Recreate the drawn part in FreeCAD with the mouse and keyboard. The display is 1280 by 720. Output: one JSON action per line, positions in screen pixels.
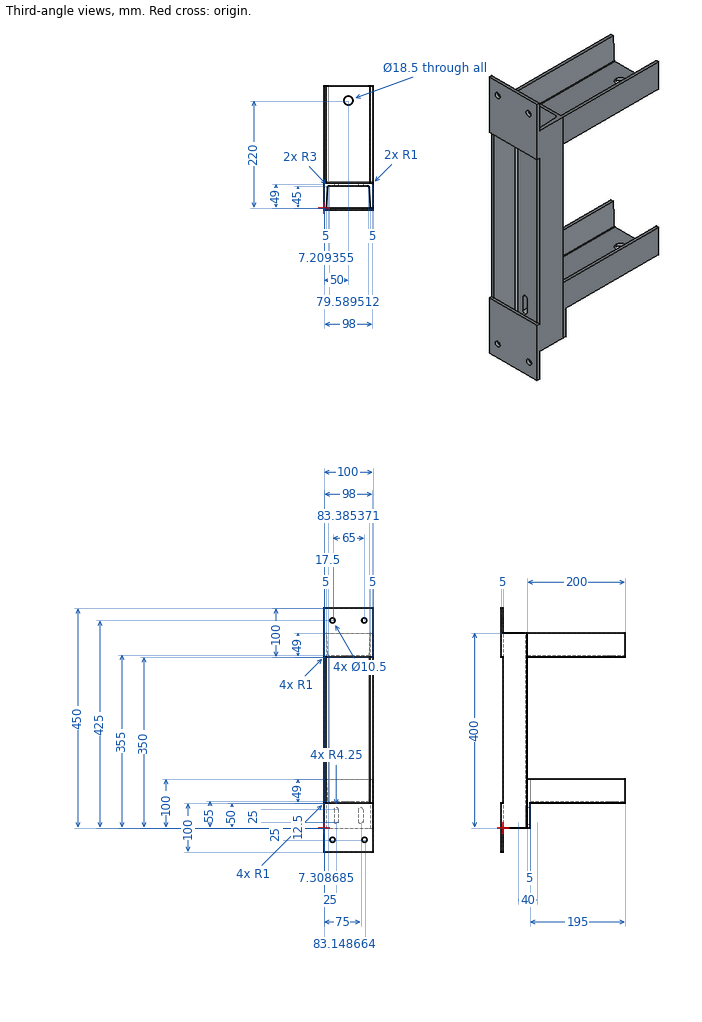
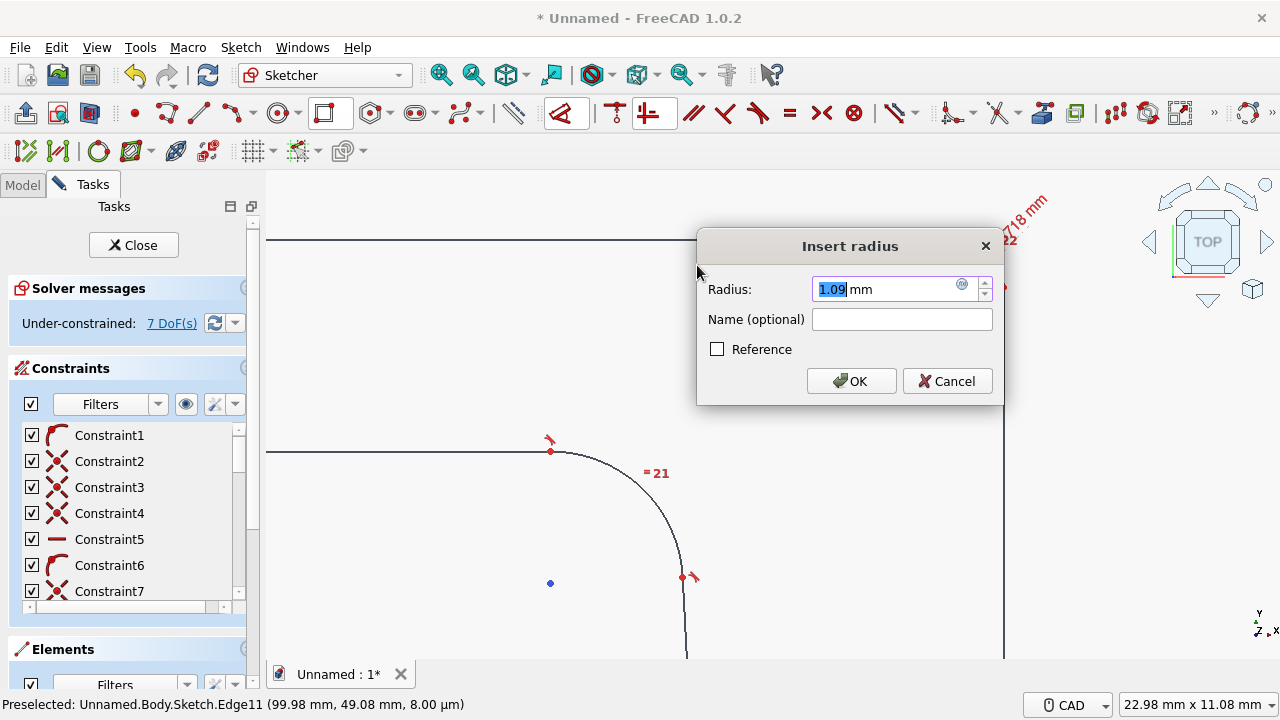
{"action": "type", "text": "1"}
{"action": "key", "text": "Return"}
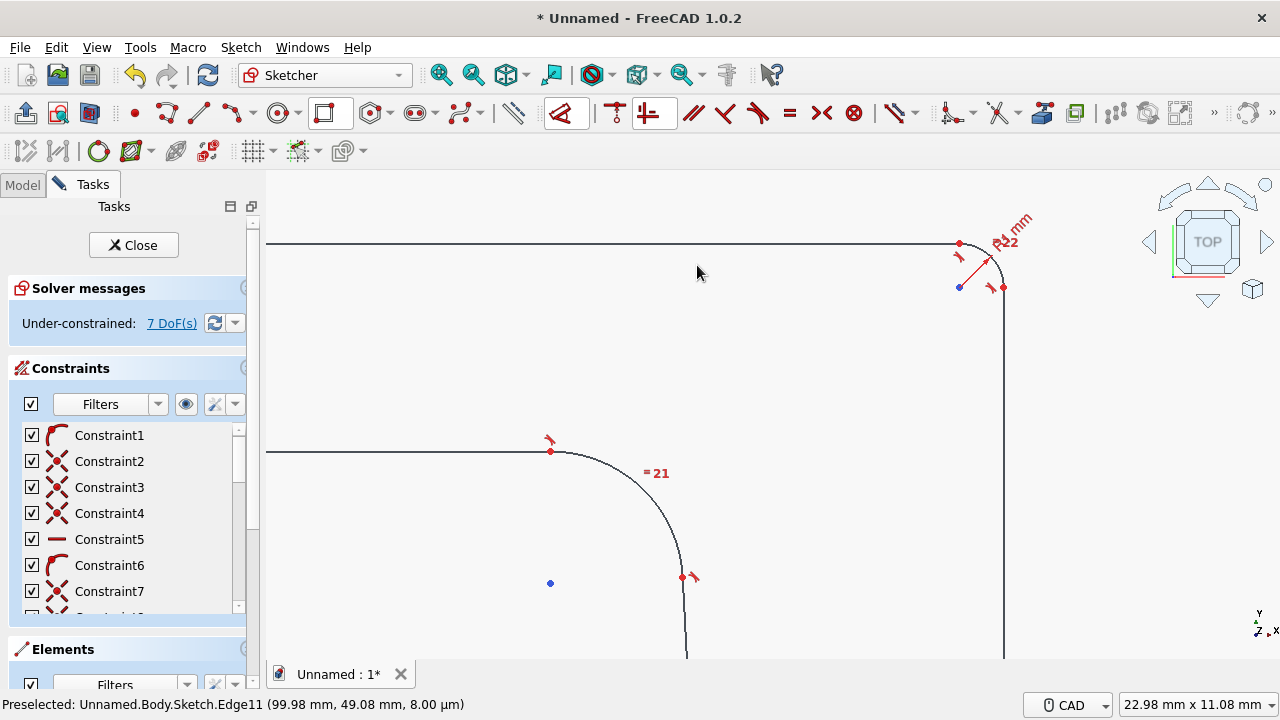
{"action": "scroll", "coordinate": [1003, 271], "scroll_direction": "down", "scroll_amount": 10}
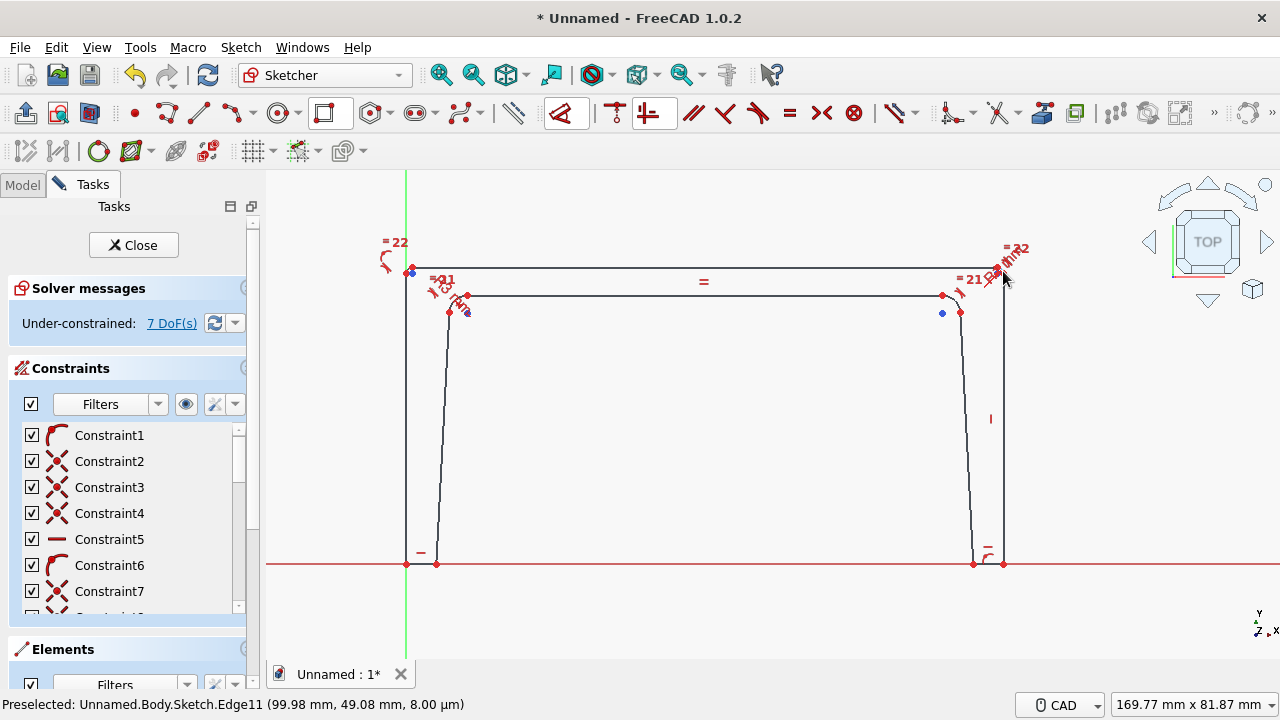
{"action": "scroll", "coordinate": [415, 564], "scroll_direction": "up", "scroll_amount": 3}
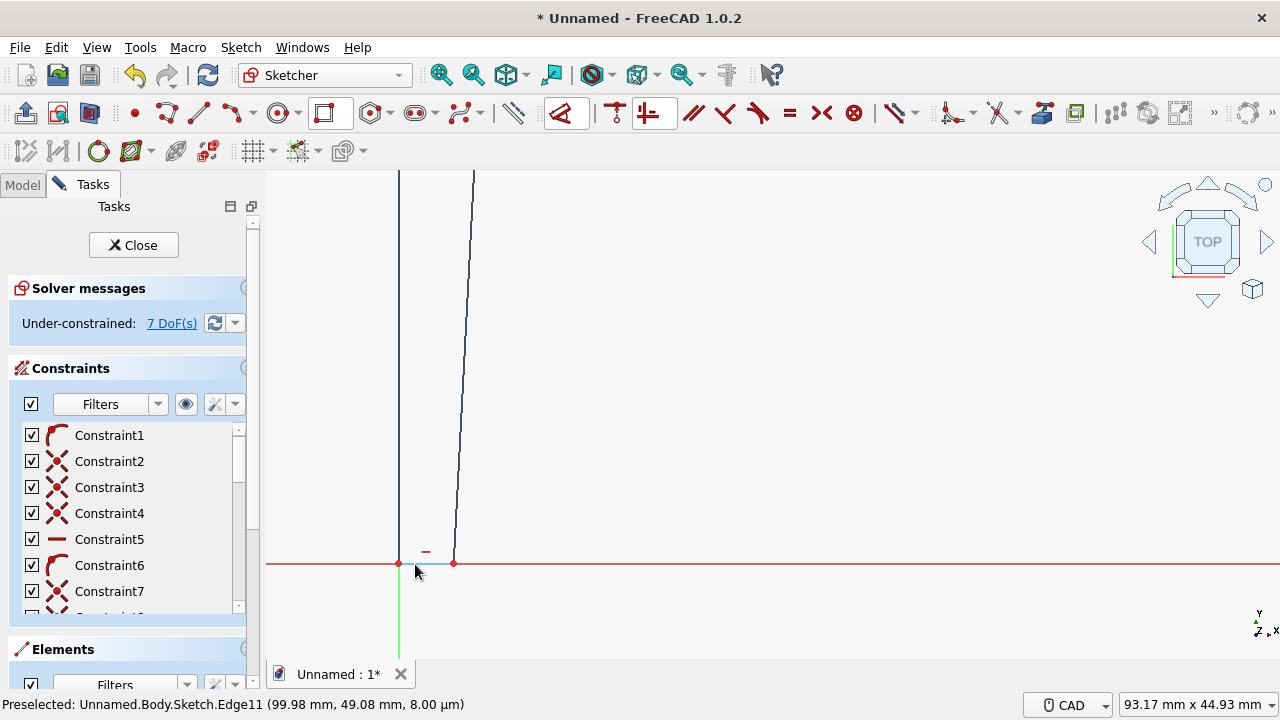
{"action": "left_click", "coordinate": [415, 564]}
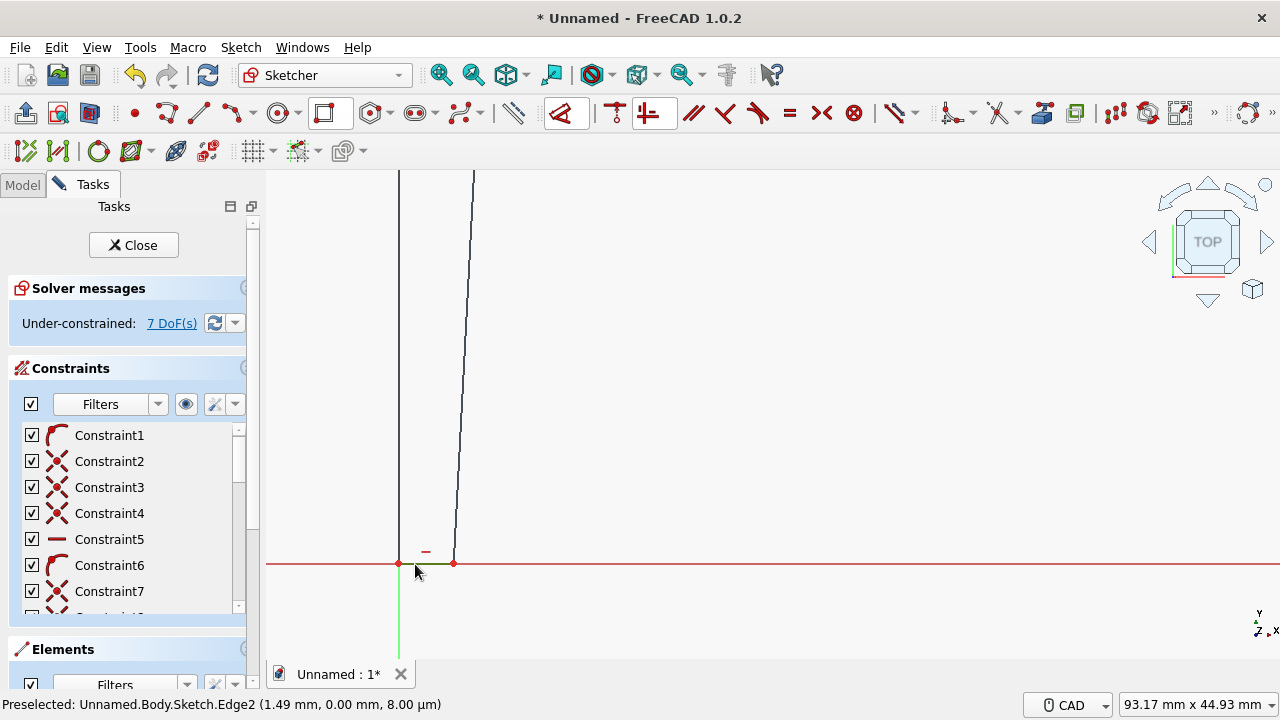
{"action": "key", "text": "l"}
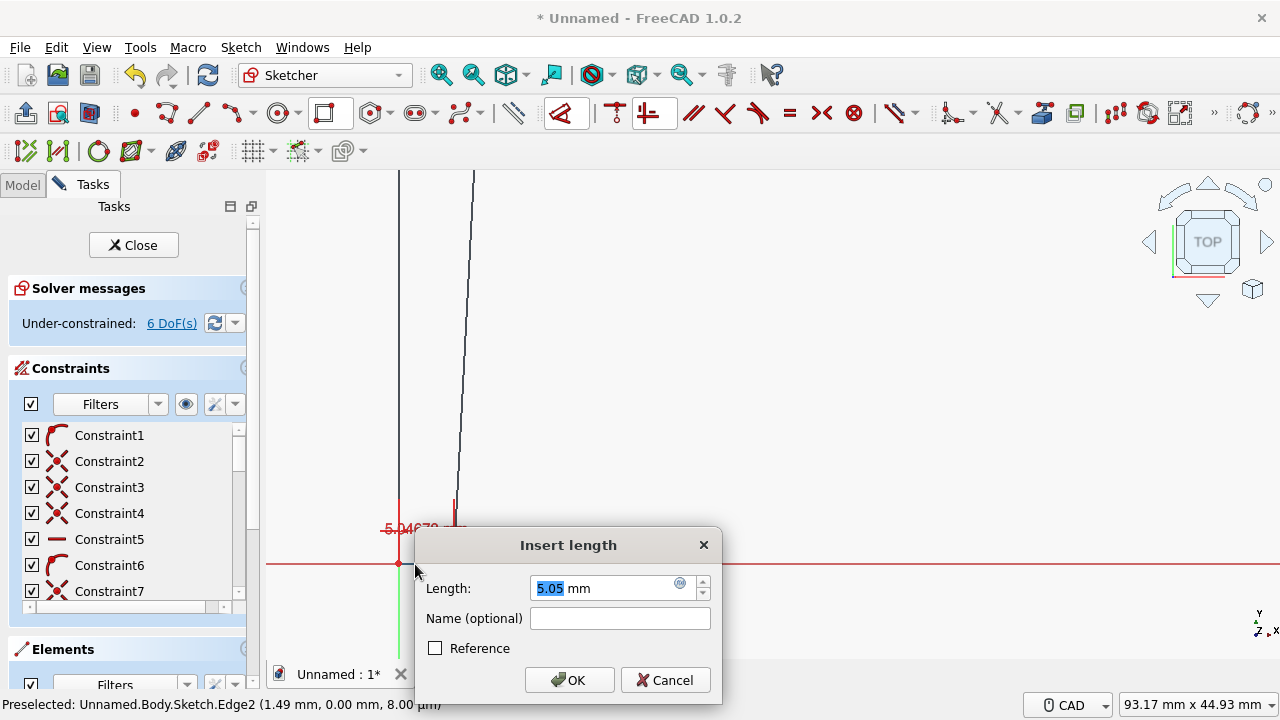
{"action": "type", "text": "5"}
{"action": "key", "text": "Return"}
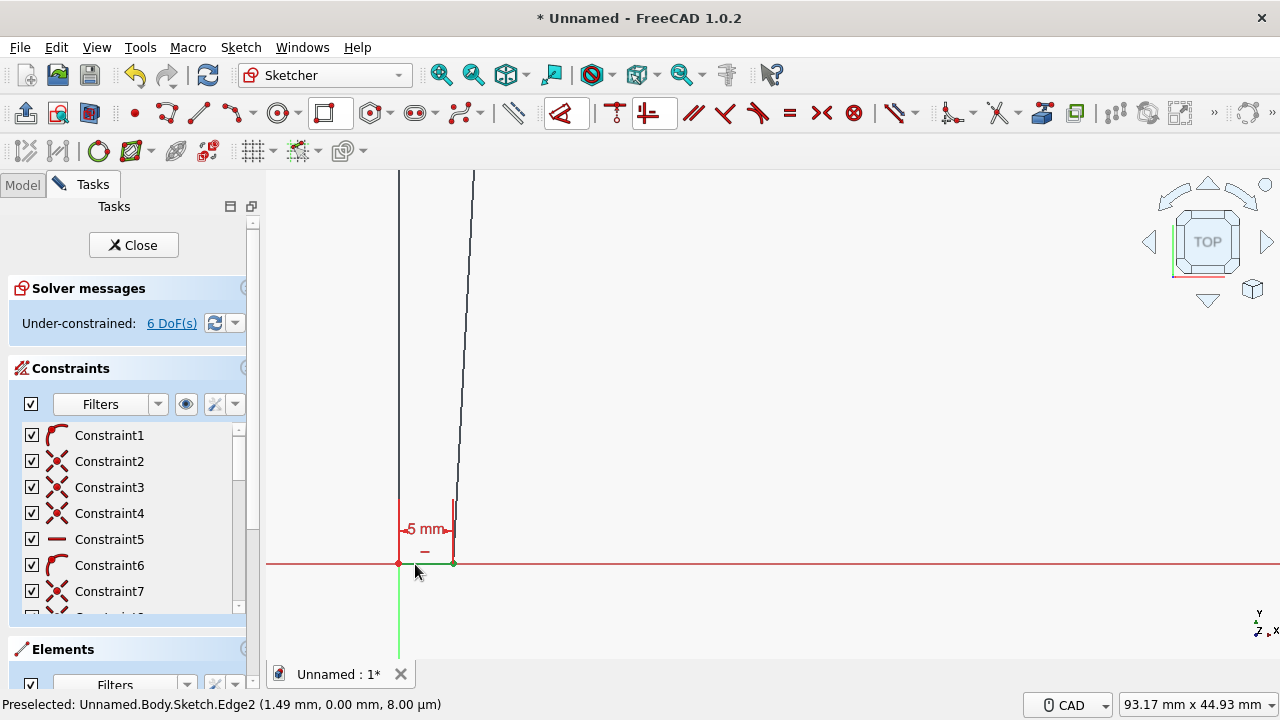
{"action": "scroll", "coordinate": [415, 564], "scroll_direction": "down", "scroll_amount": 3}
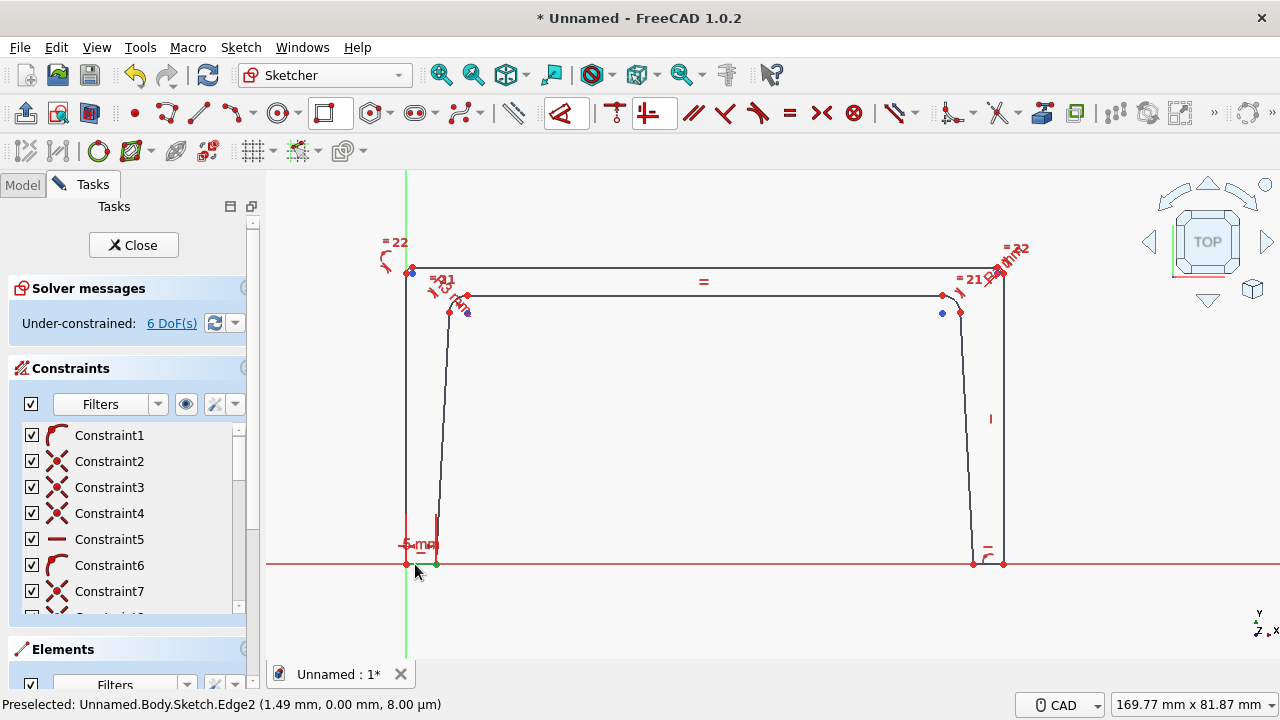
{"action": "scroll", "coordinate": [982, 564], "scroll_direction": "up", "scroll_amount": 3}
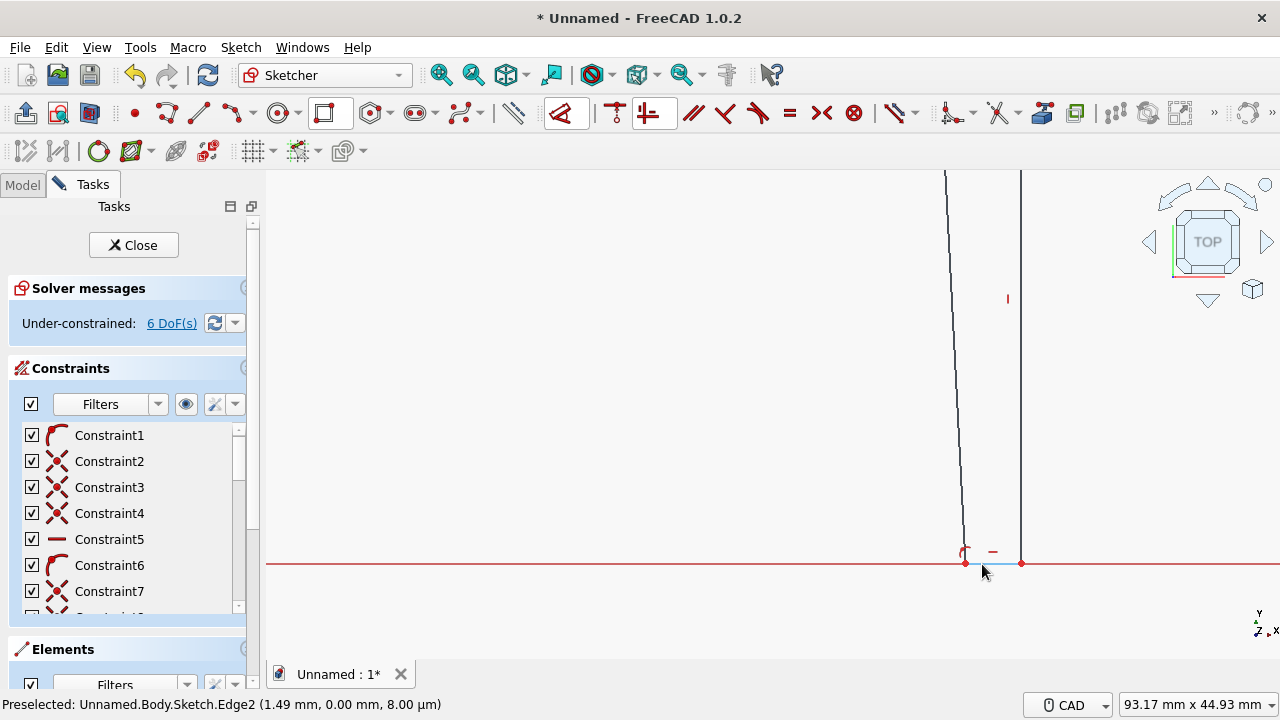
{"action": "left_click", "coordinate": [982, 564]}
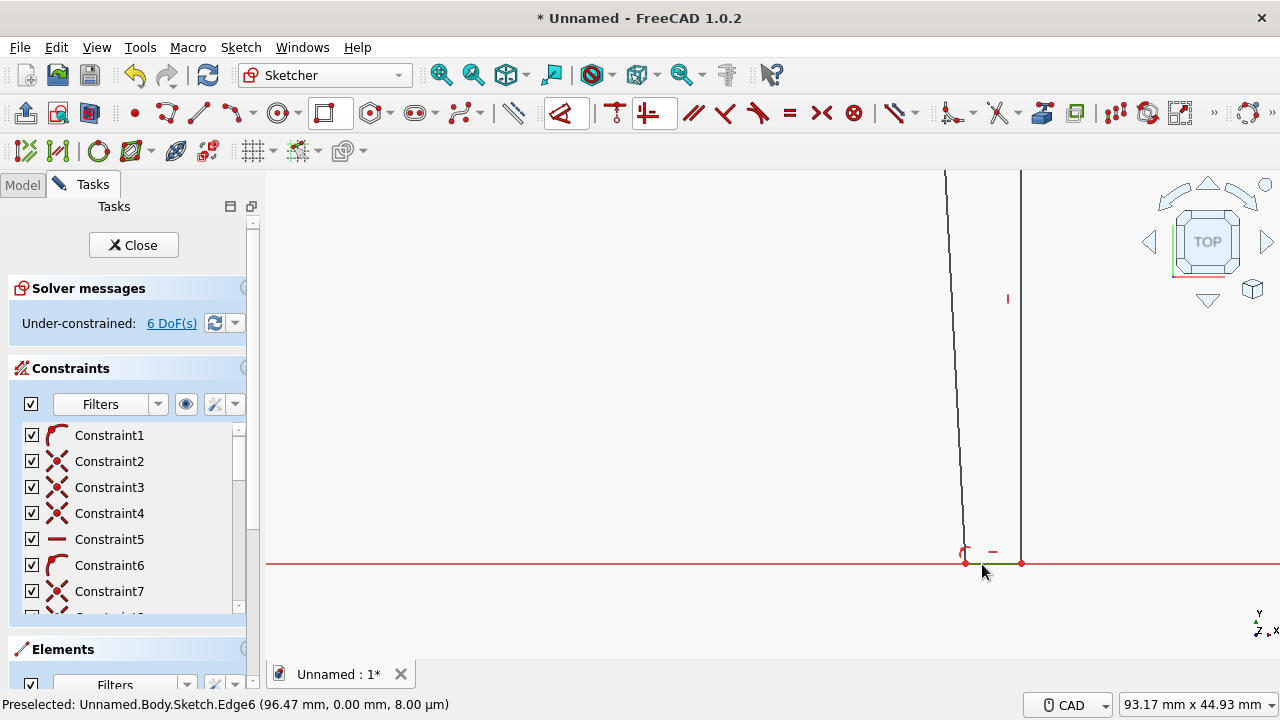
{"action": "left_click", "coordinate": [584, 114]}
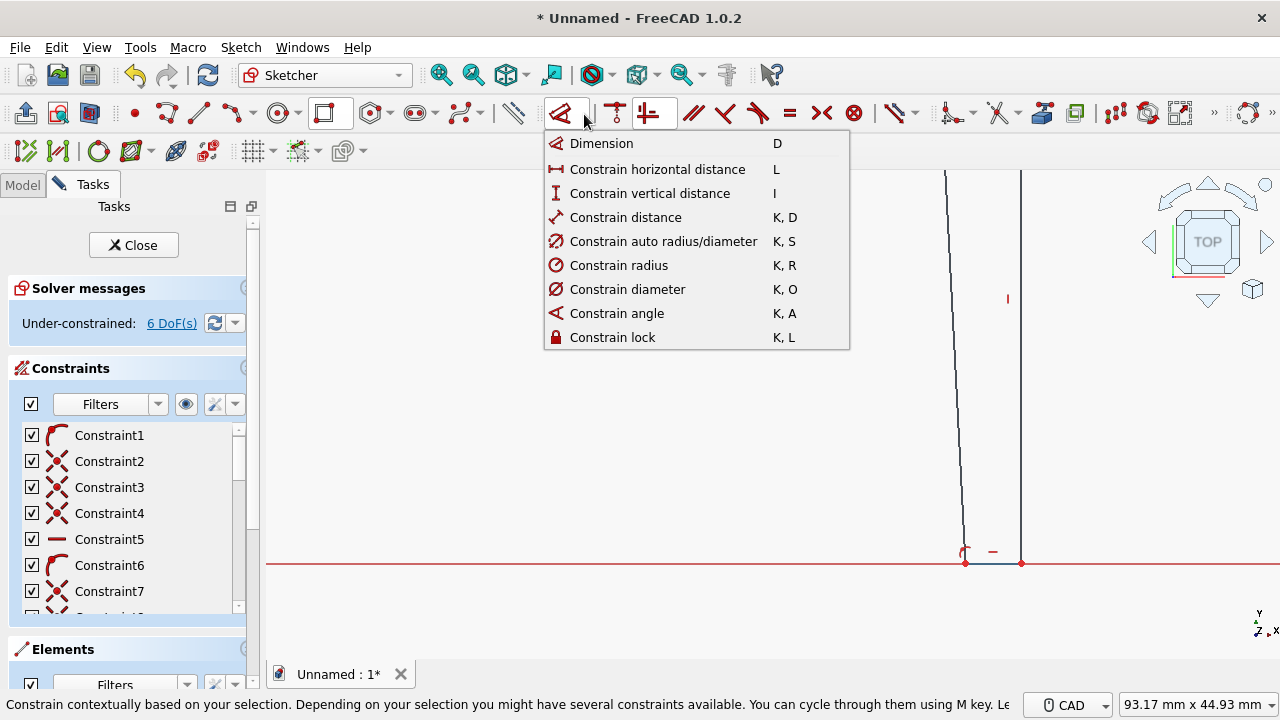
{"action": "left_click", "coordinate": [697, 169]}